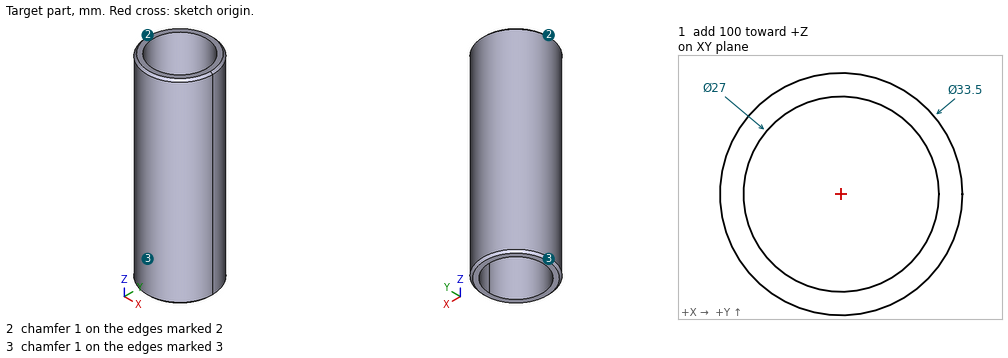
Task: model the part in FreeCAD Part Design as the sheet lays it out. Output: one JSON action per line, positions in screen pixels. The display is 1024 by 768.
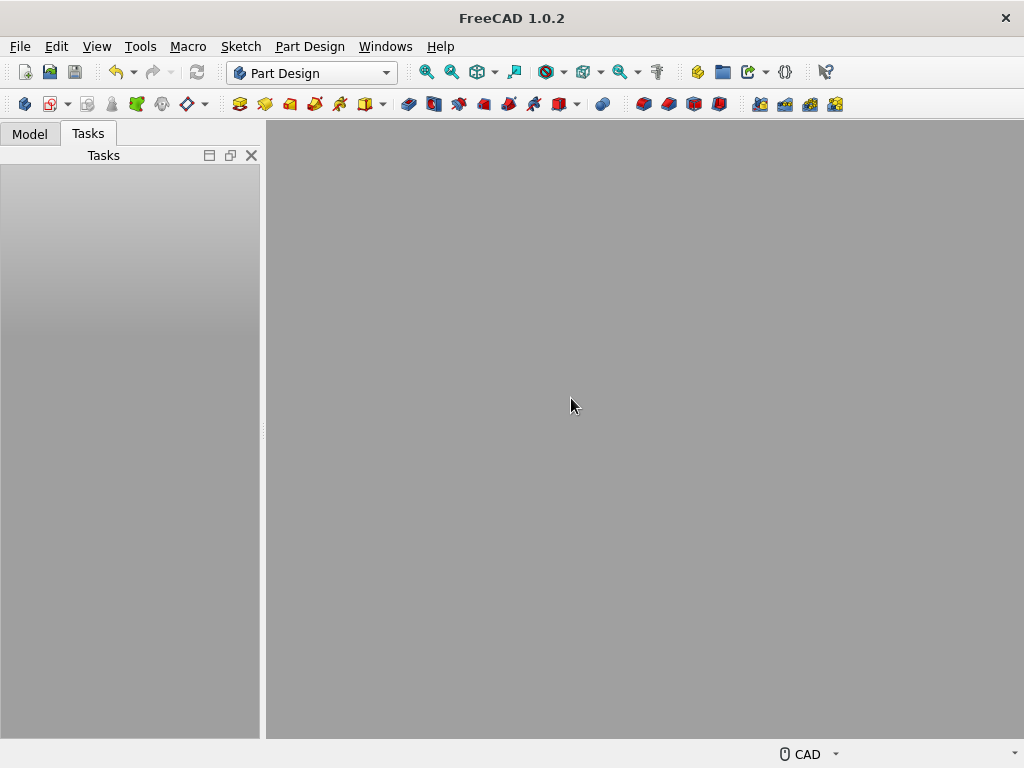
{"action": "left_click", "coordinate": [25, 72]}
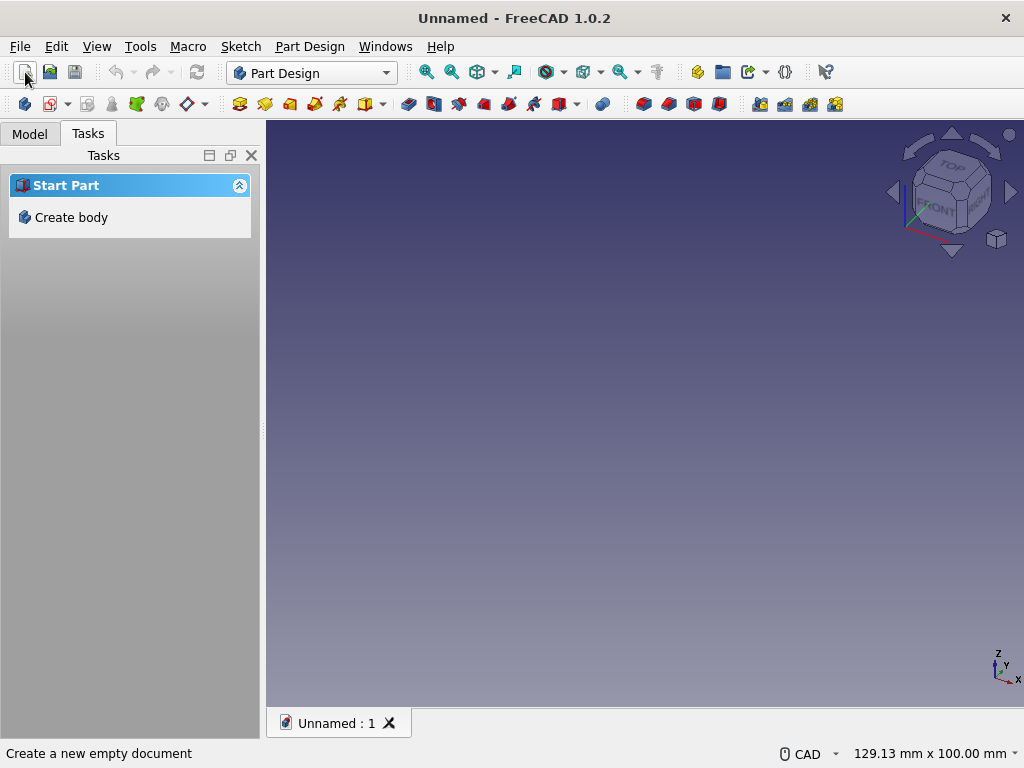
{"action": "left_click", "coordinate": [50, 104]}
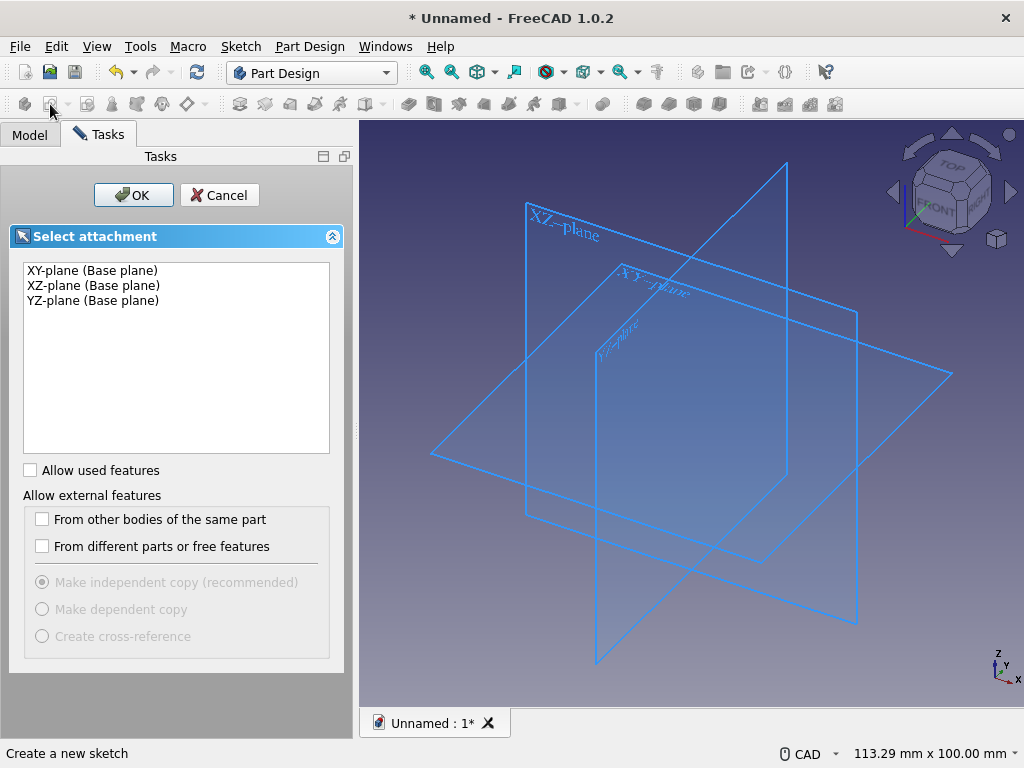
{"action": "left_click", "coordinate": [84, 270]}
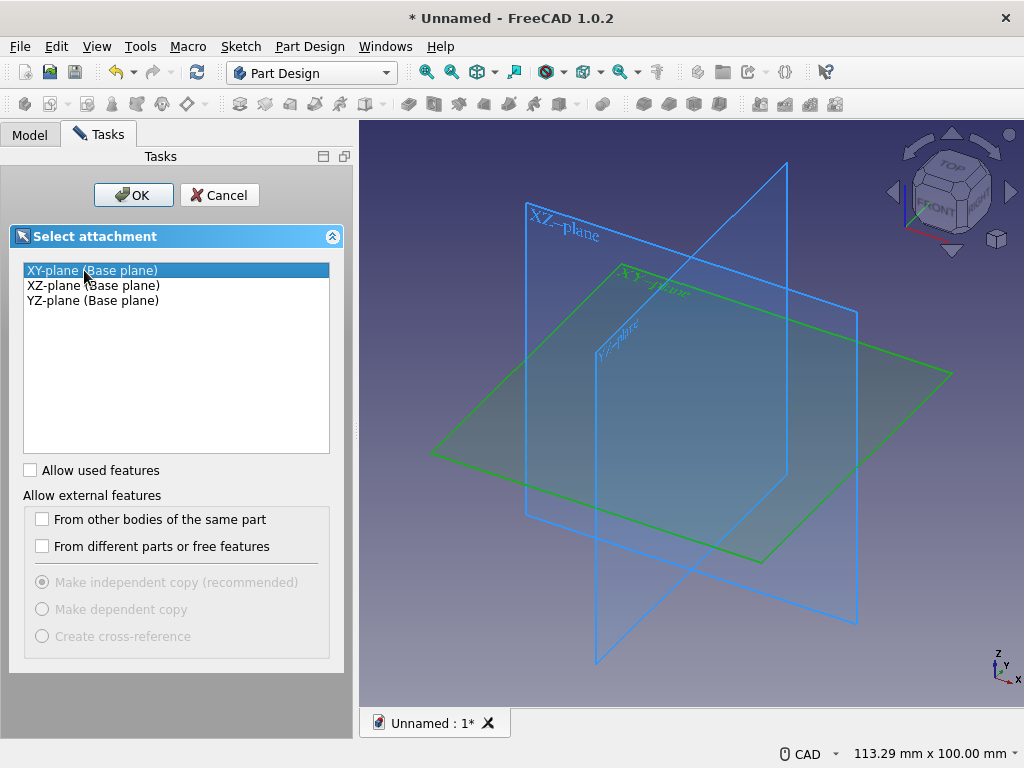
{"action": "left_click", "coordinate": [134, 195]}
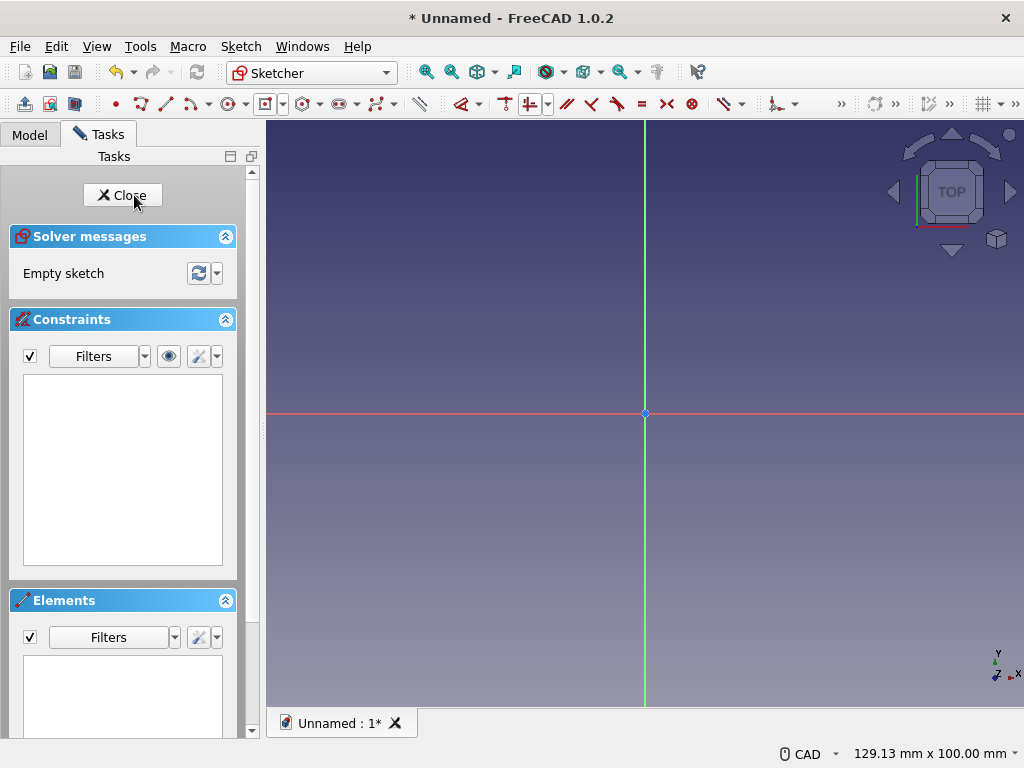
{"action": "scroll", "coordinate": [728, 414], "scroll_direction": "up", "scroll_amount": 3}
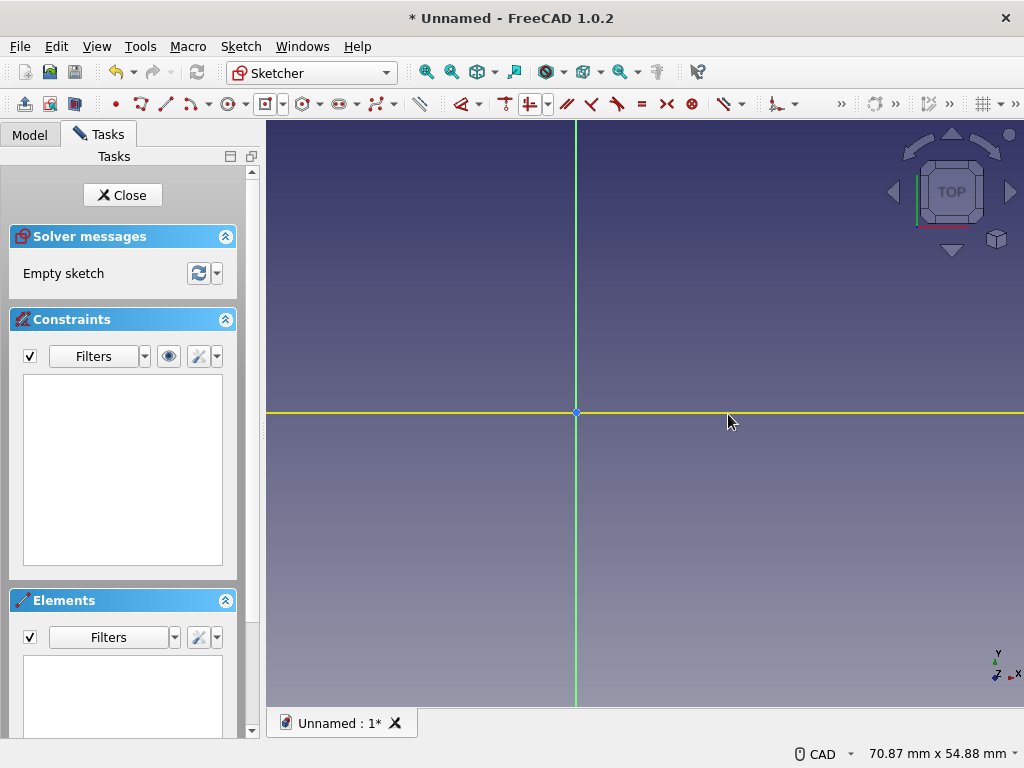
{"action": "left_click", "coordinate": [228, 104]}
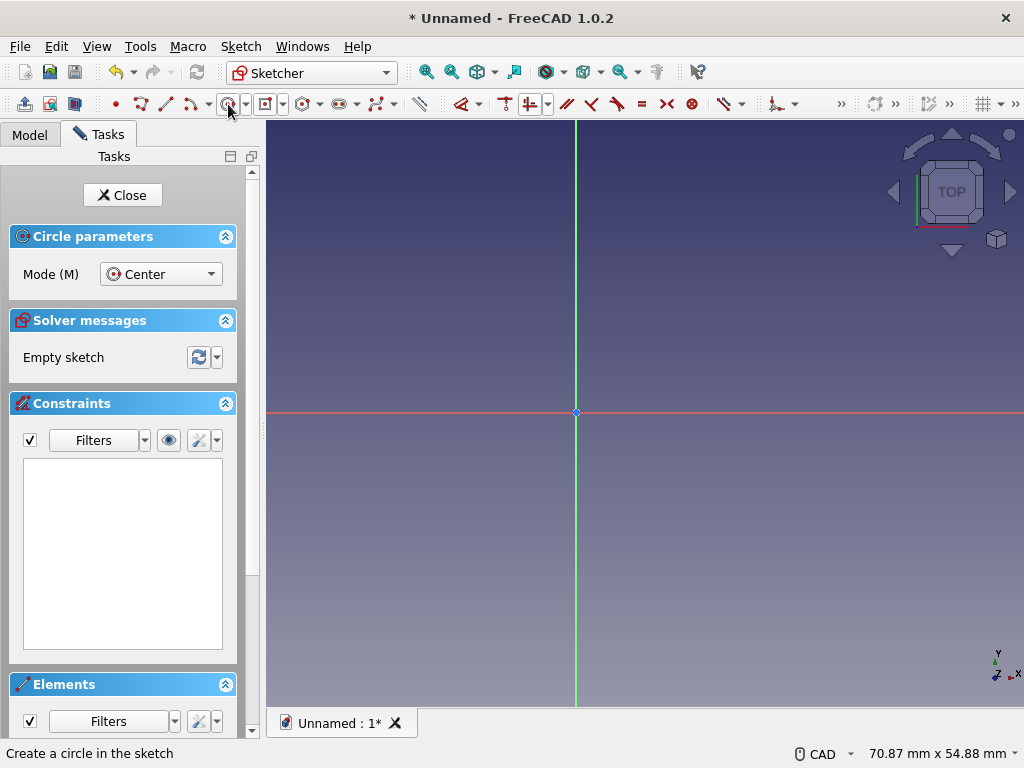
{"action": "left_click", "coordinate": [576, 413]}
{"action": "left_click", "coordinate": [703, 286]}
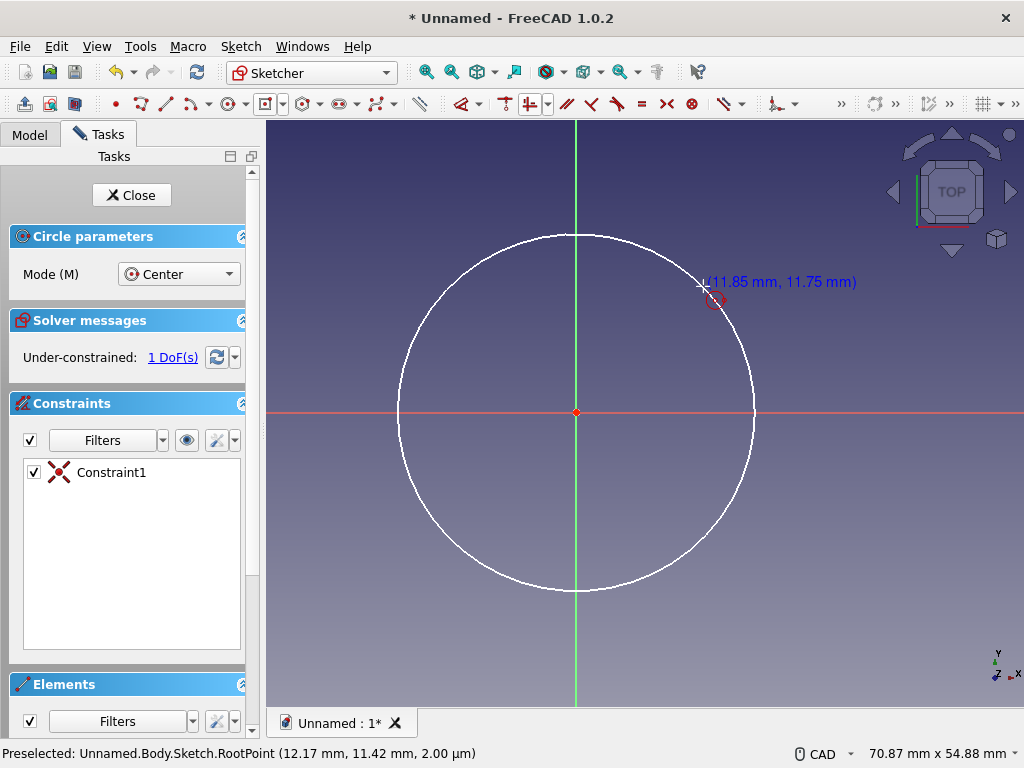
{"action": "left_click", "coordinate": [576, 413]}
{"action": "left_click", "coordinate": [678, 311]}
{"action": "key", "text": "Escape"}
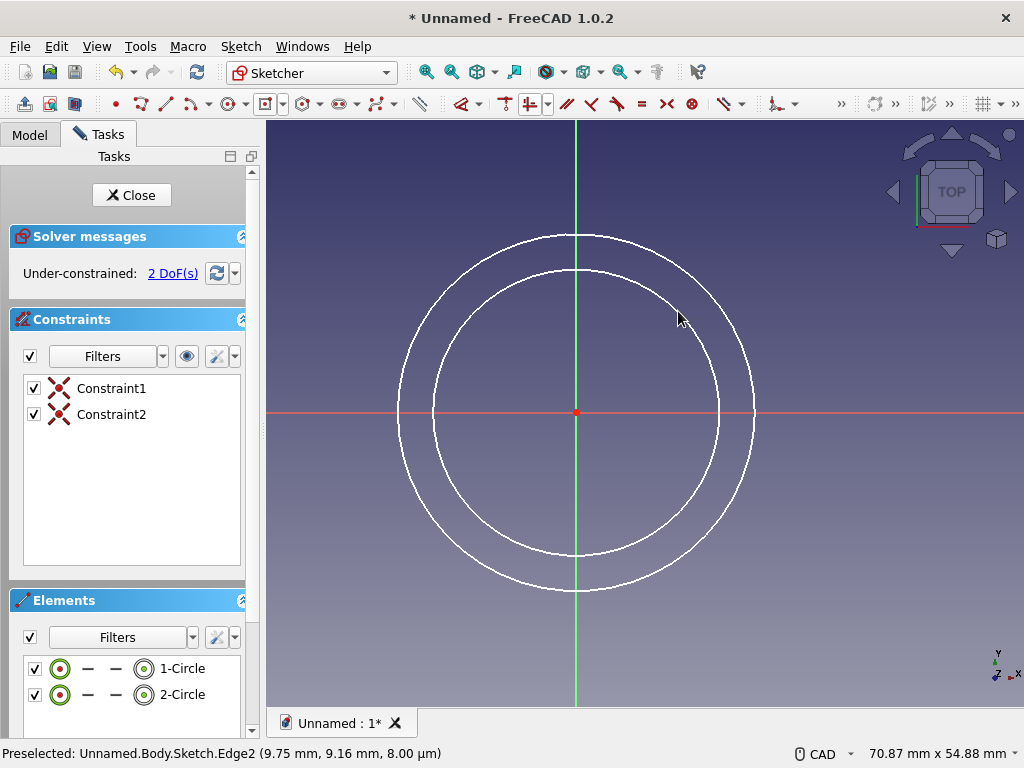
{"action": "left_click", "coordinate": [460, 104]}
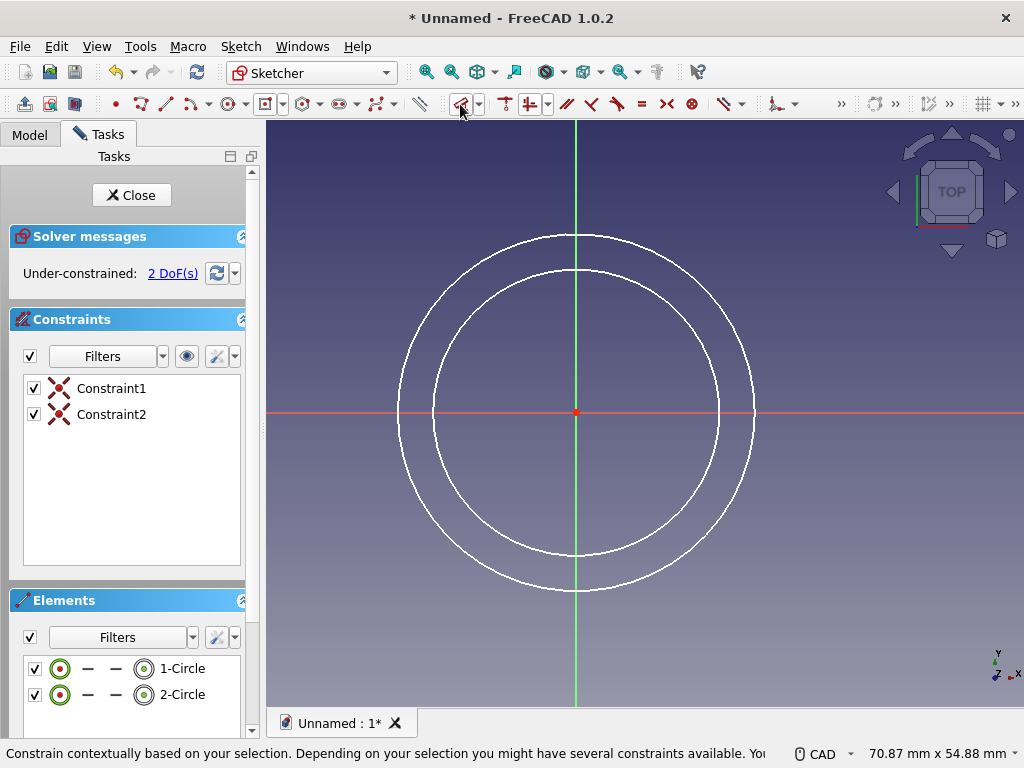
{"action": "left_click", "coordinate": [702, 286]}
{"action": "left_click", "coordinate": [725, 263]}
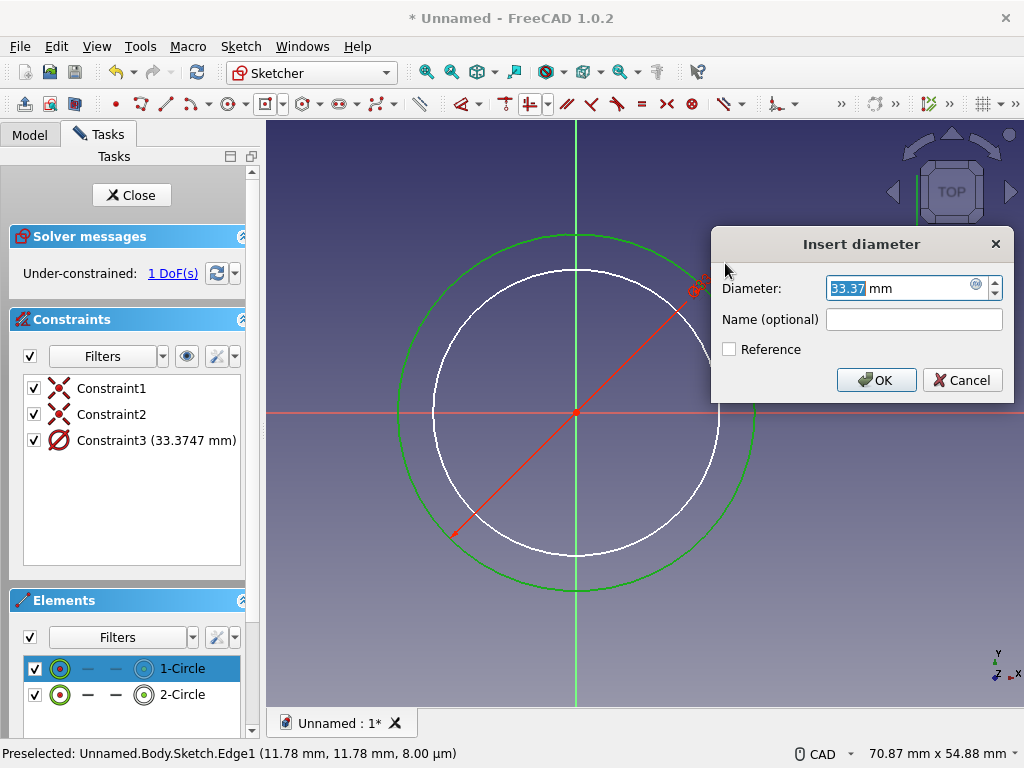
{"action": "type", "text": "33.5"}
{"action": "key", "text": "Return"}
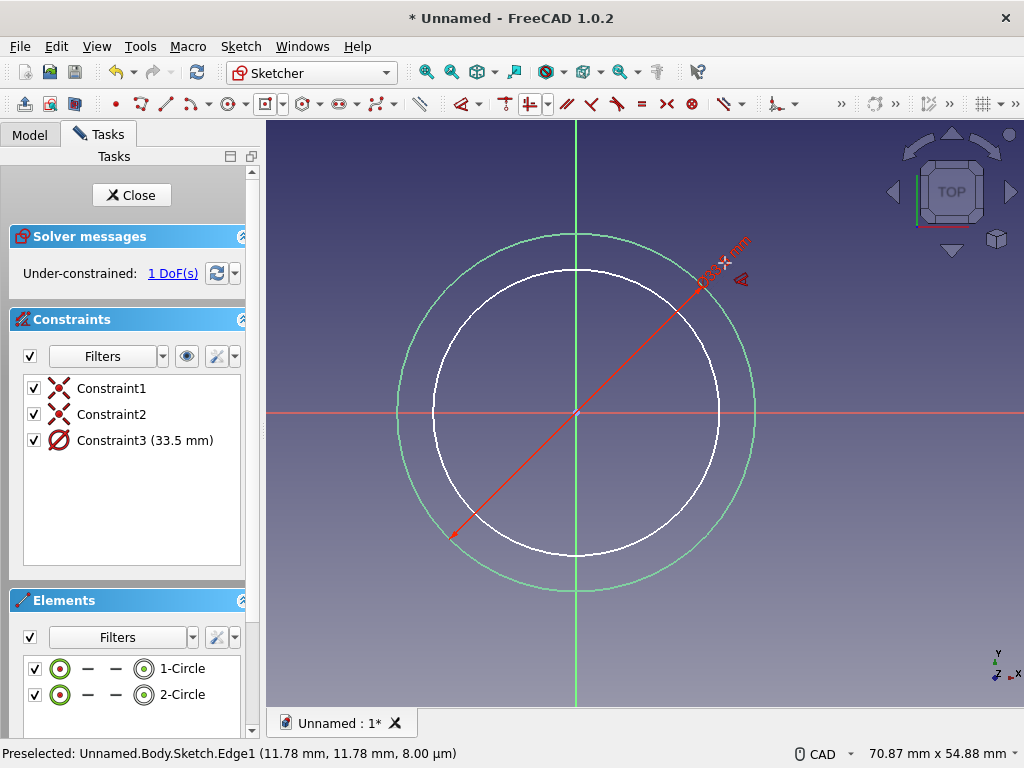
{"action": "left_click", "coordinate": [677, 311]}
{"action": "left_click", "coordinate": [766, 356]}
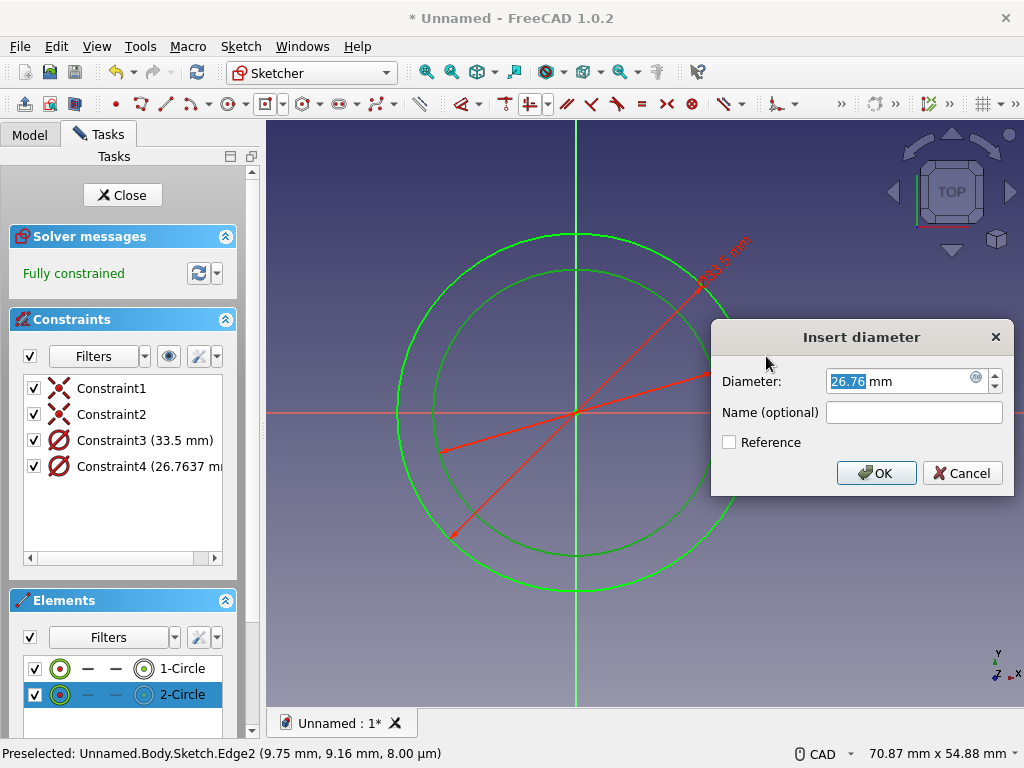
{"action": "type", "text": "27"}
{"action": "key", "text": "Return"}
{"action": "key", "text": "Escape"}